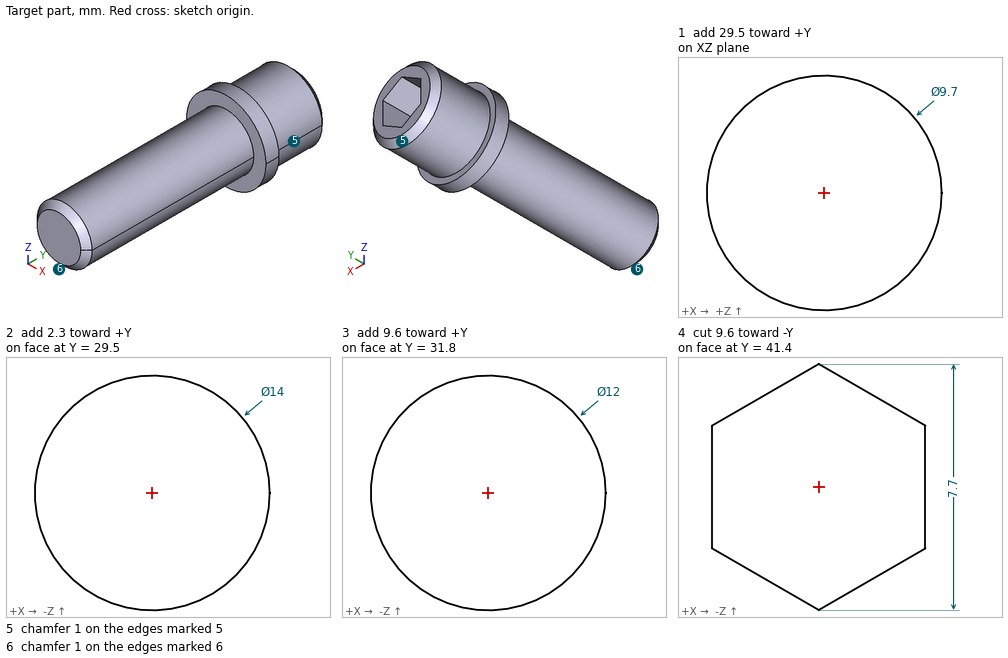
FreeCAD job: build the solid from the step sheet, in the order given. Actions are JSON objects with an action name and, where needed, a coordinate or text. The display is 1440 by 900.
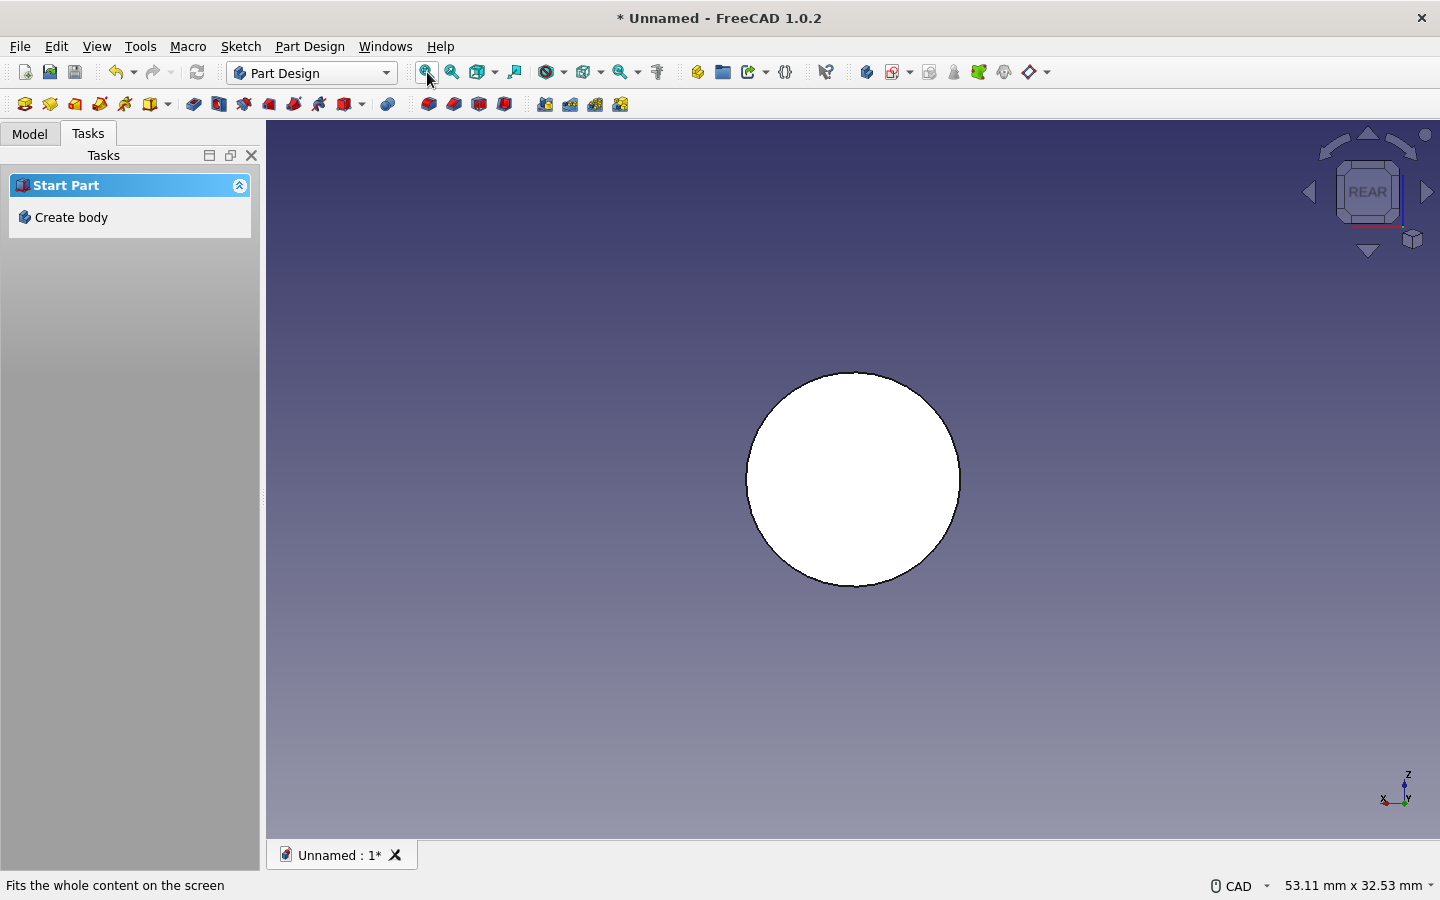
{"action": "left_click", "coordinate": [853, 479]}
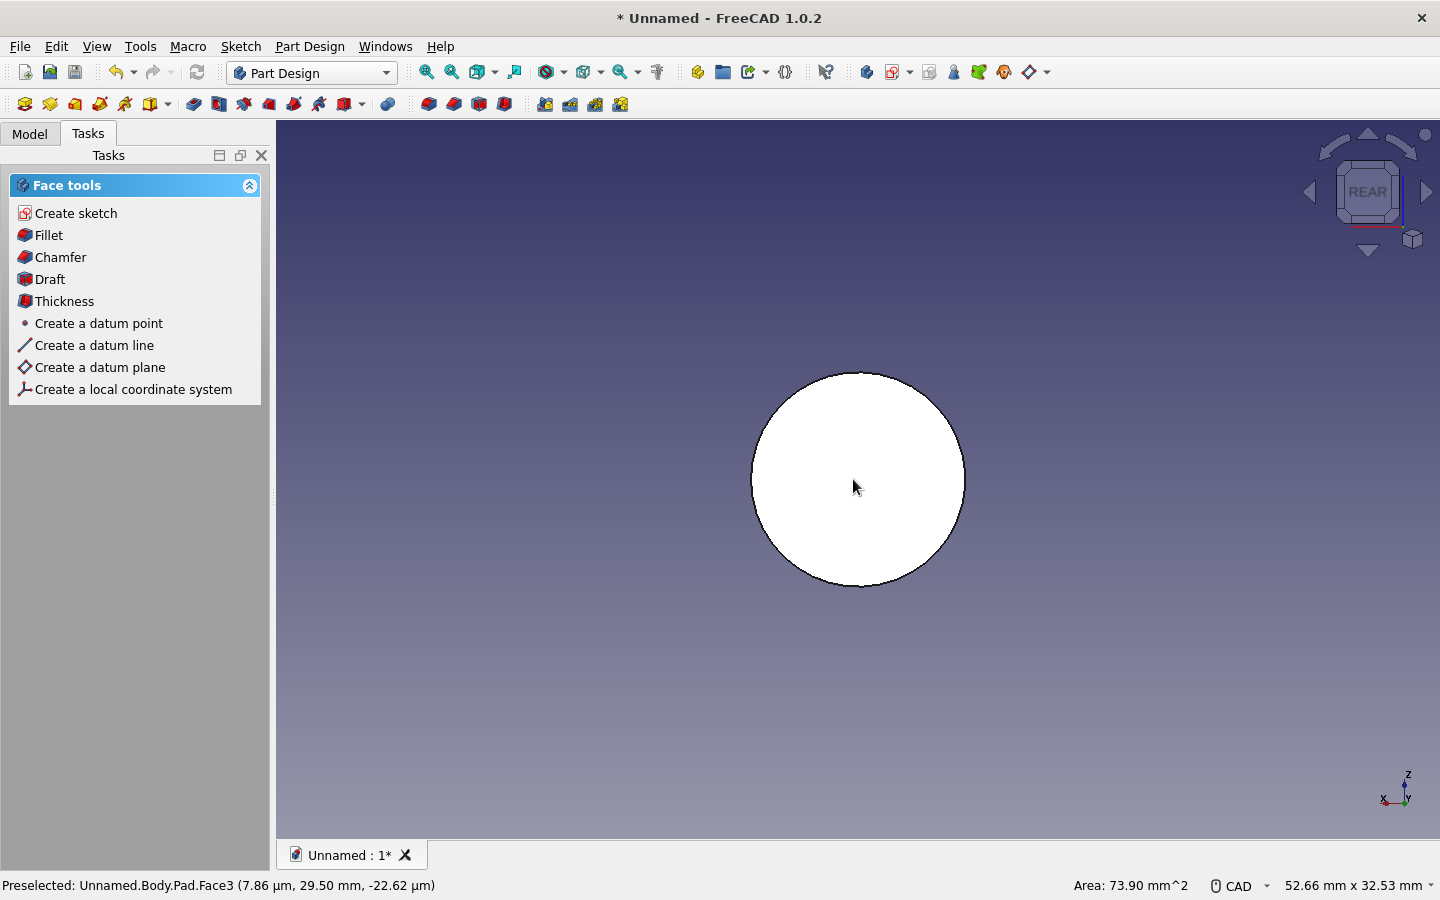
{"action": "left_click", "coordinate": [892, 72]}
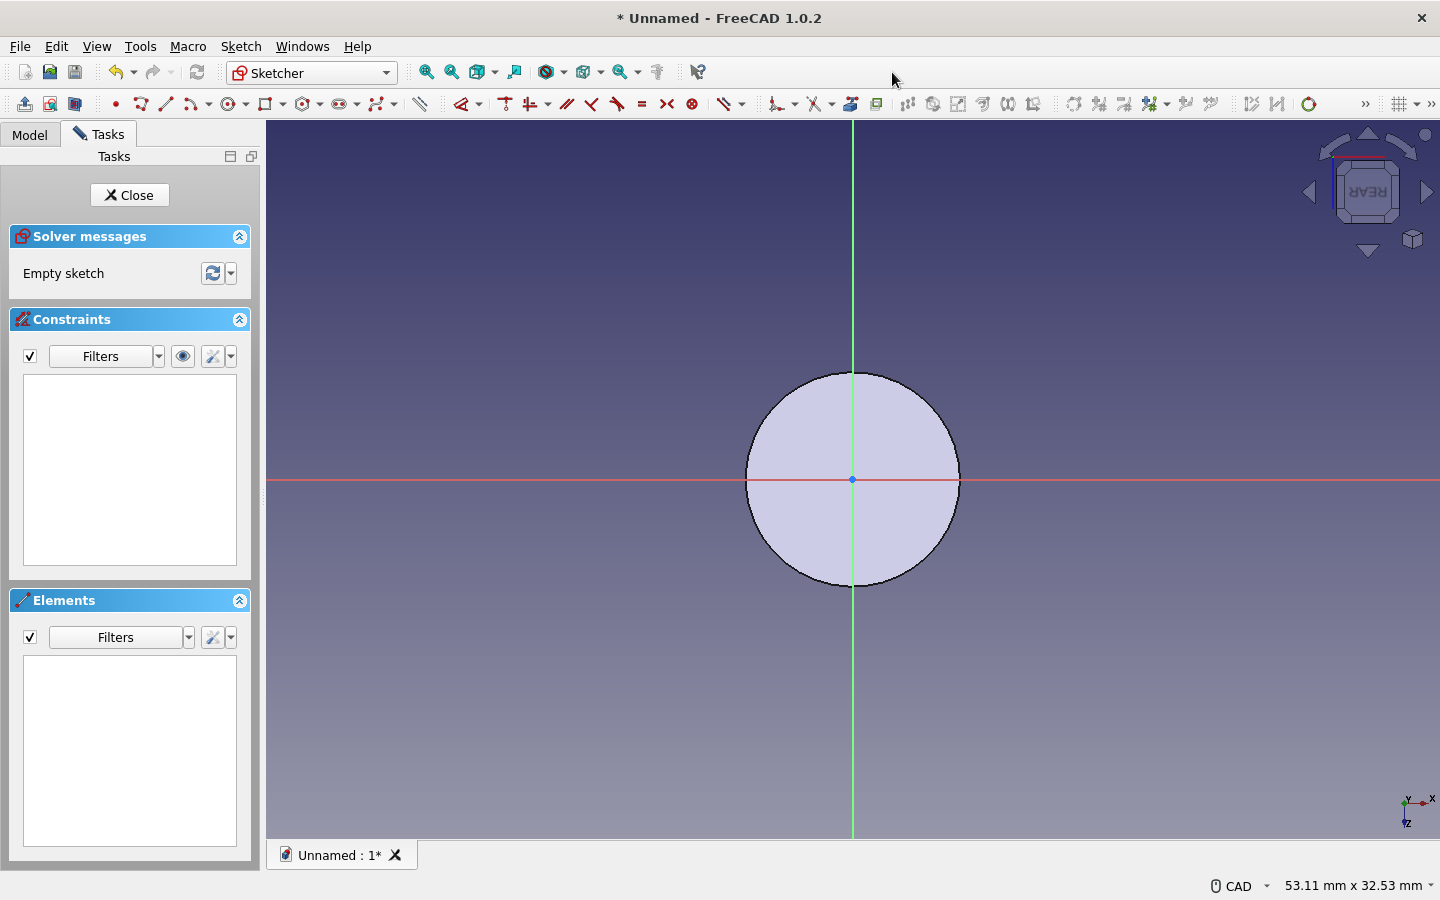
{"action": "scroll", "coordinate": [992, 479], "scroll_direction": "up", "scroll_amount": 2}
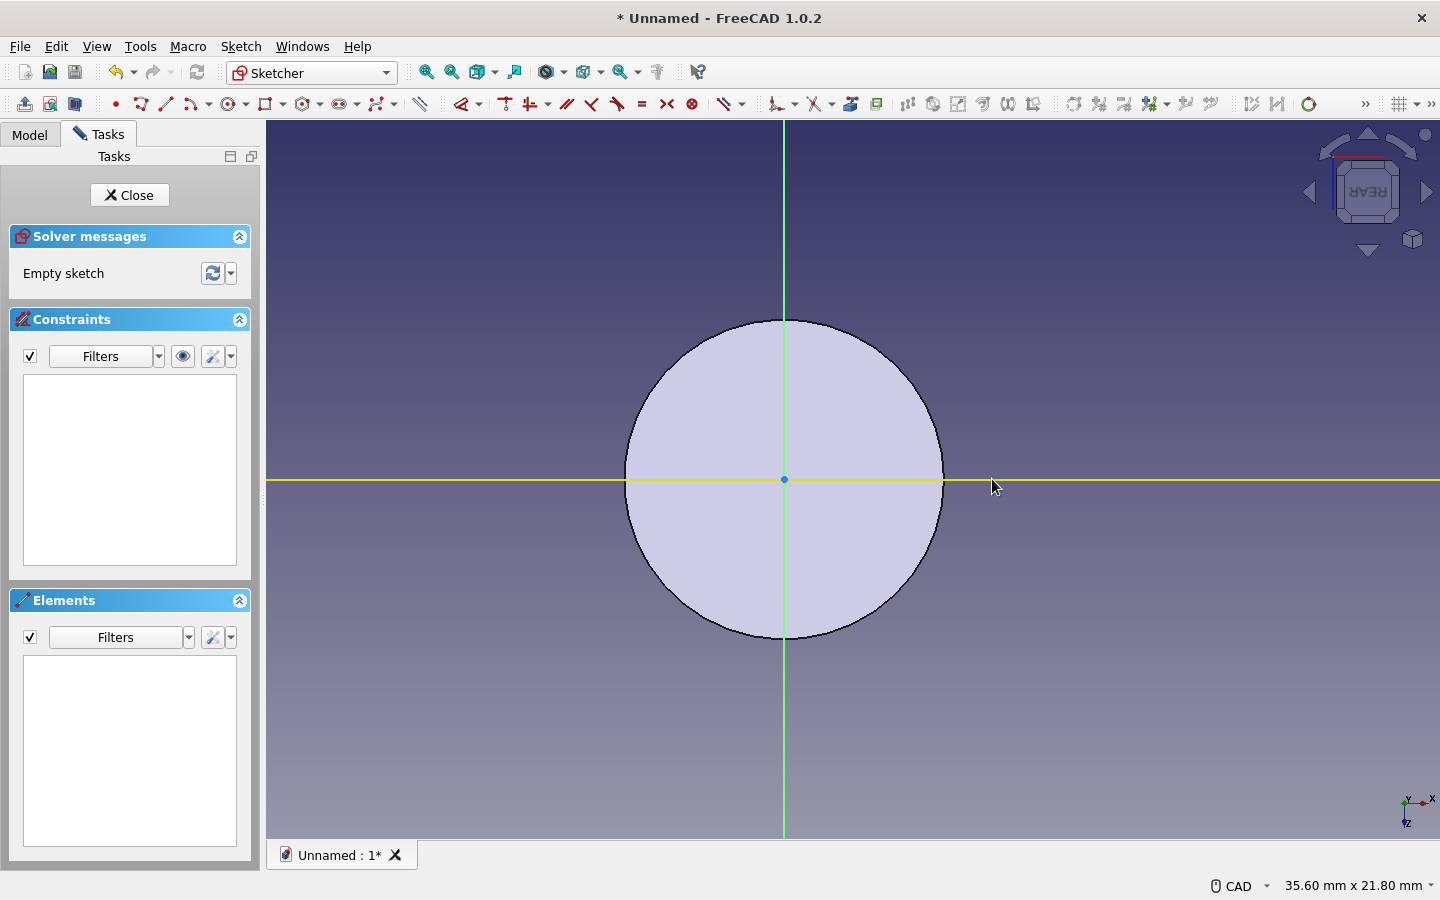
{"action": "left_click", "coordinate": [228, 104]}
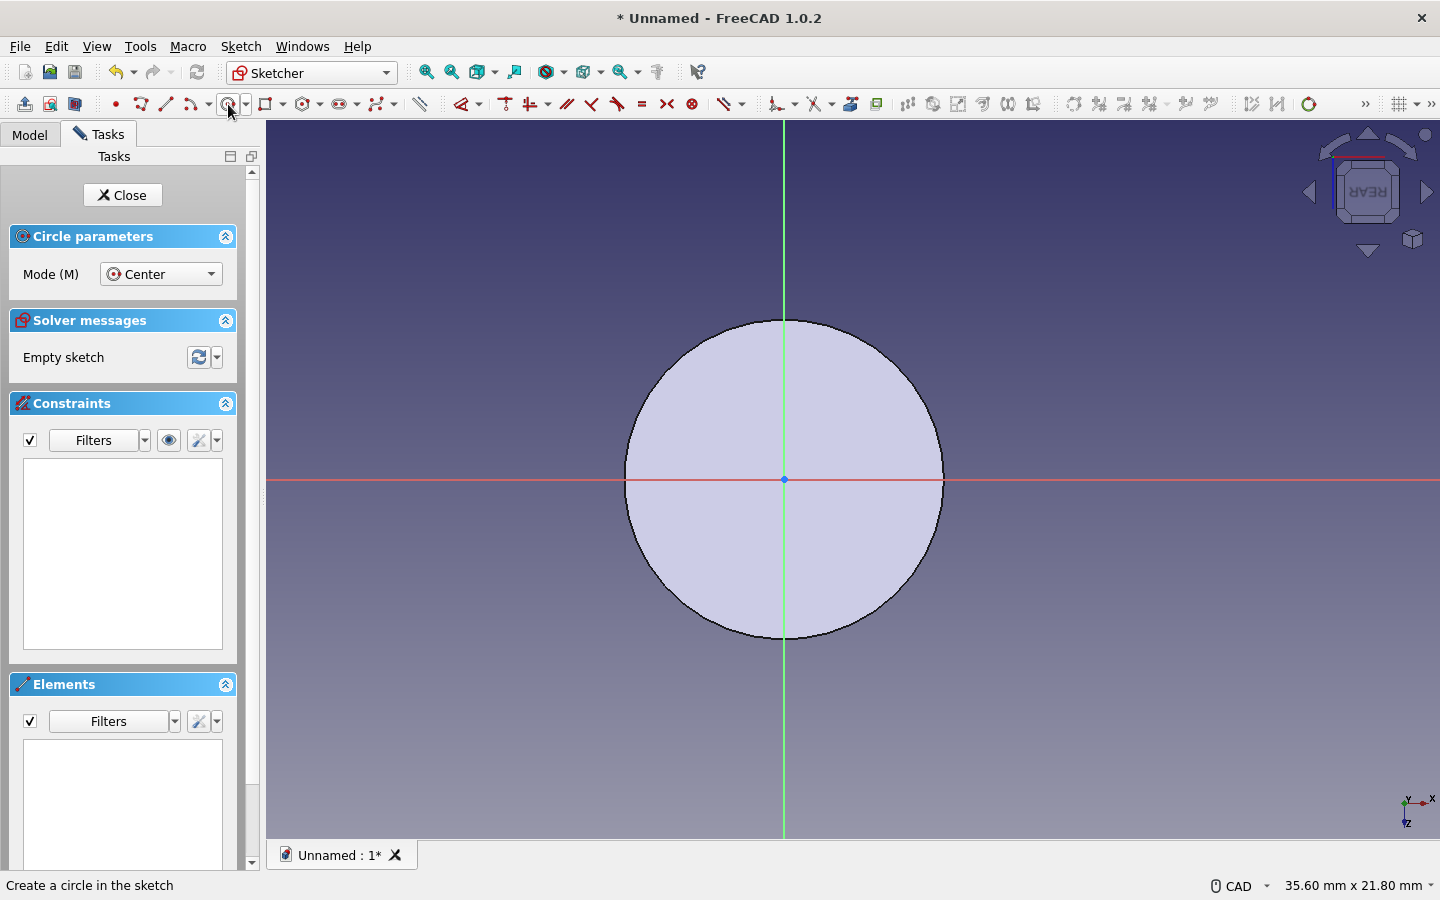
{"action": "left_click", "coordinate": [784, 479]}
{"action": "mouse_move", "coordinate": [947, 316]}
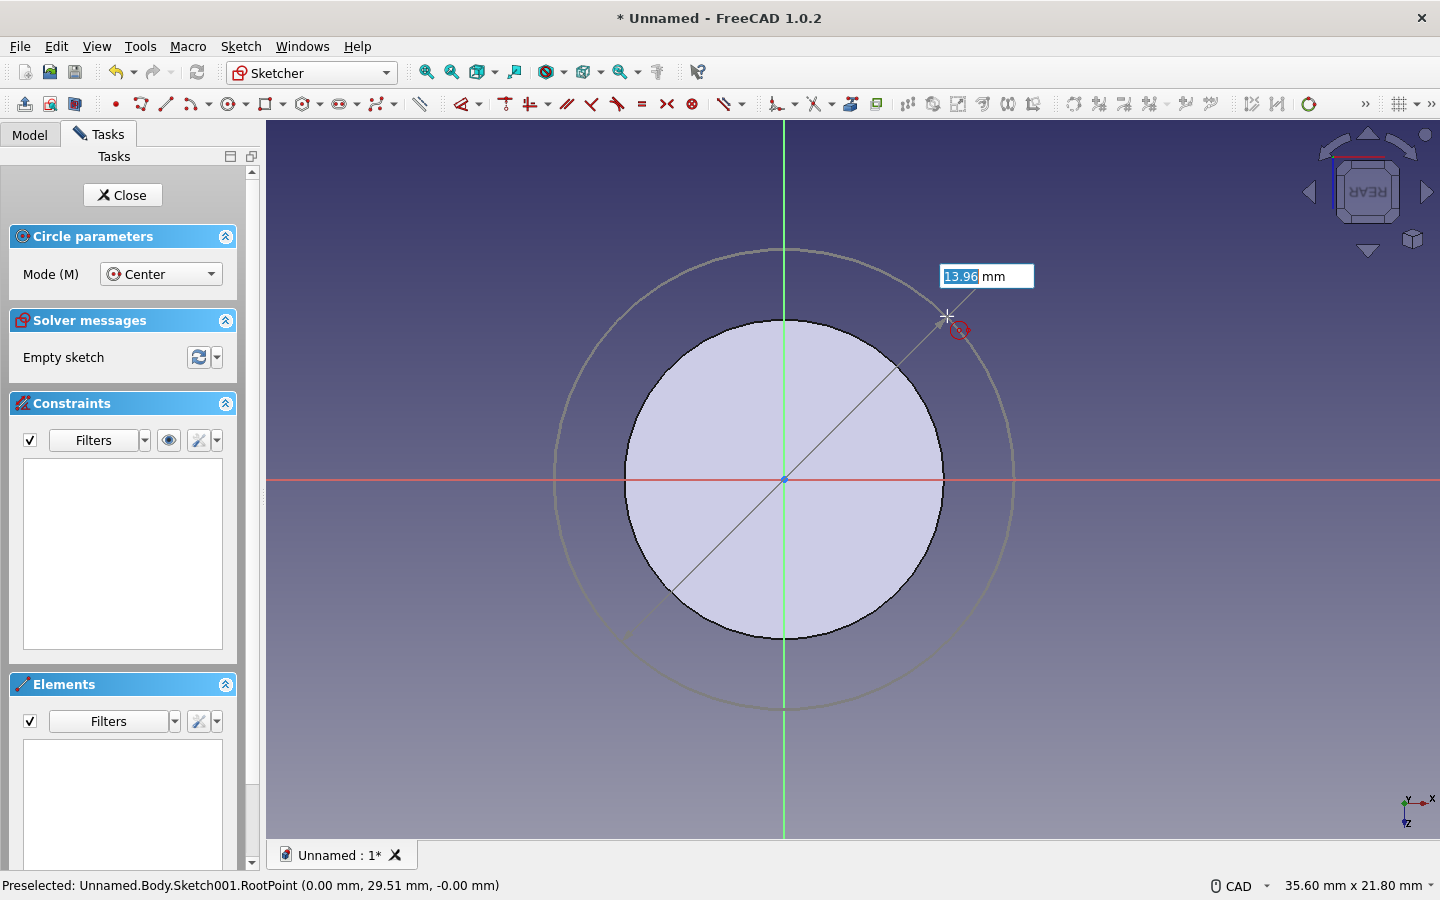
{"action": "type", "text": "14"}
{"action": "key", "text": "Return"}
{"action": "key", "text": "Escape"}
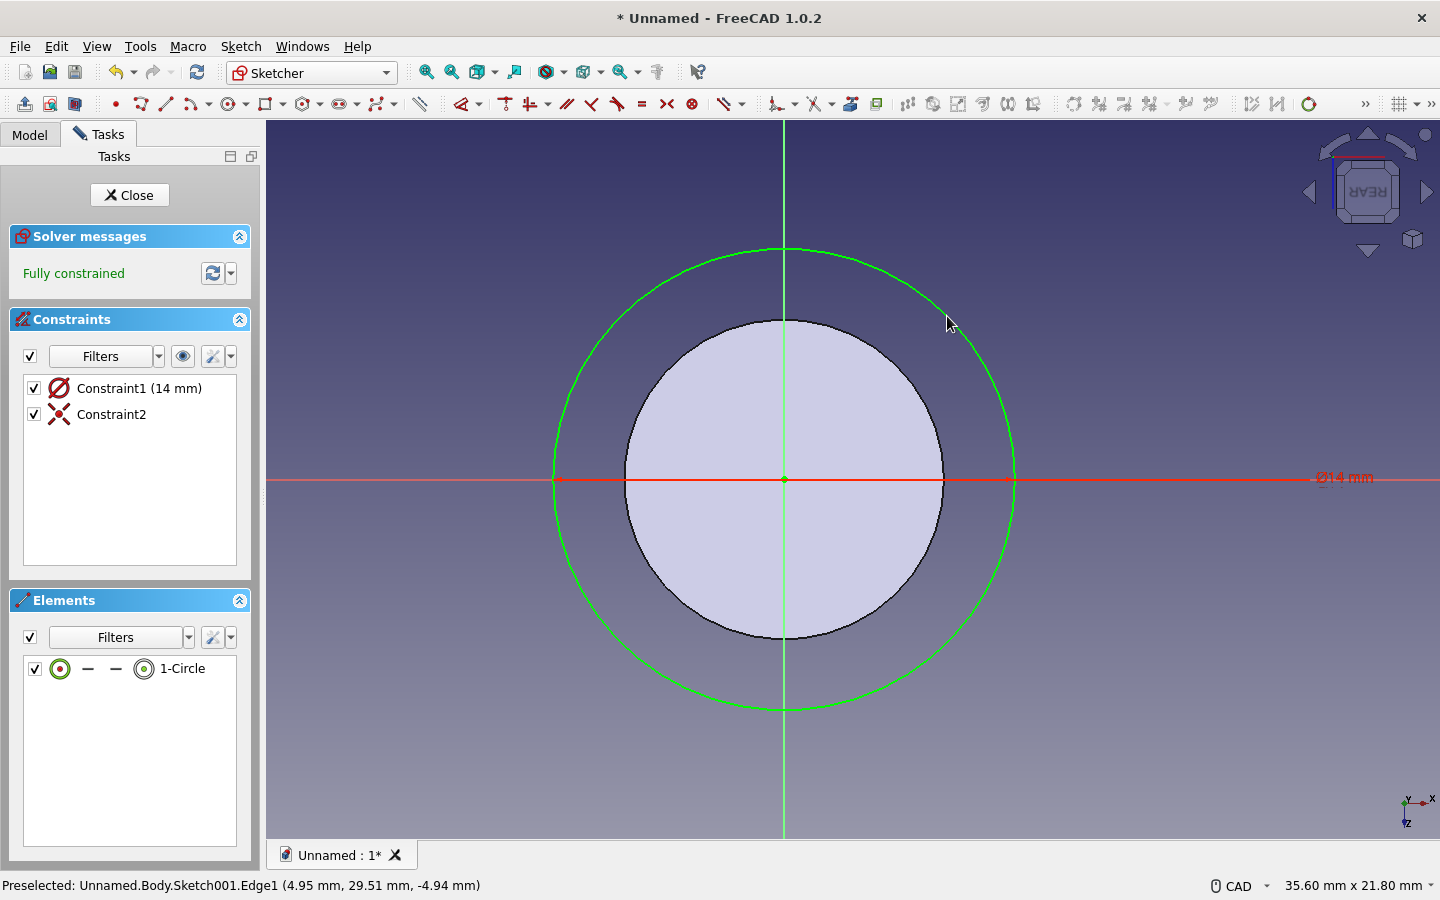
{"action": "left_click", "coordinate": [130, 195]}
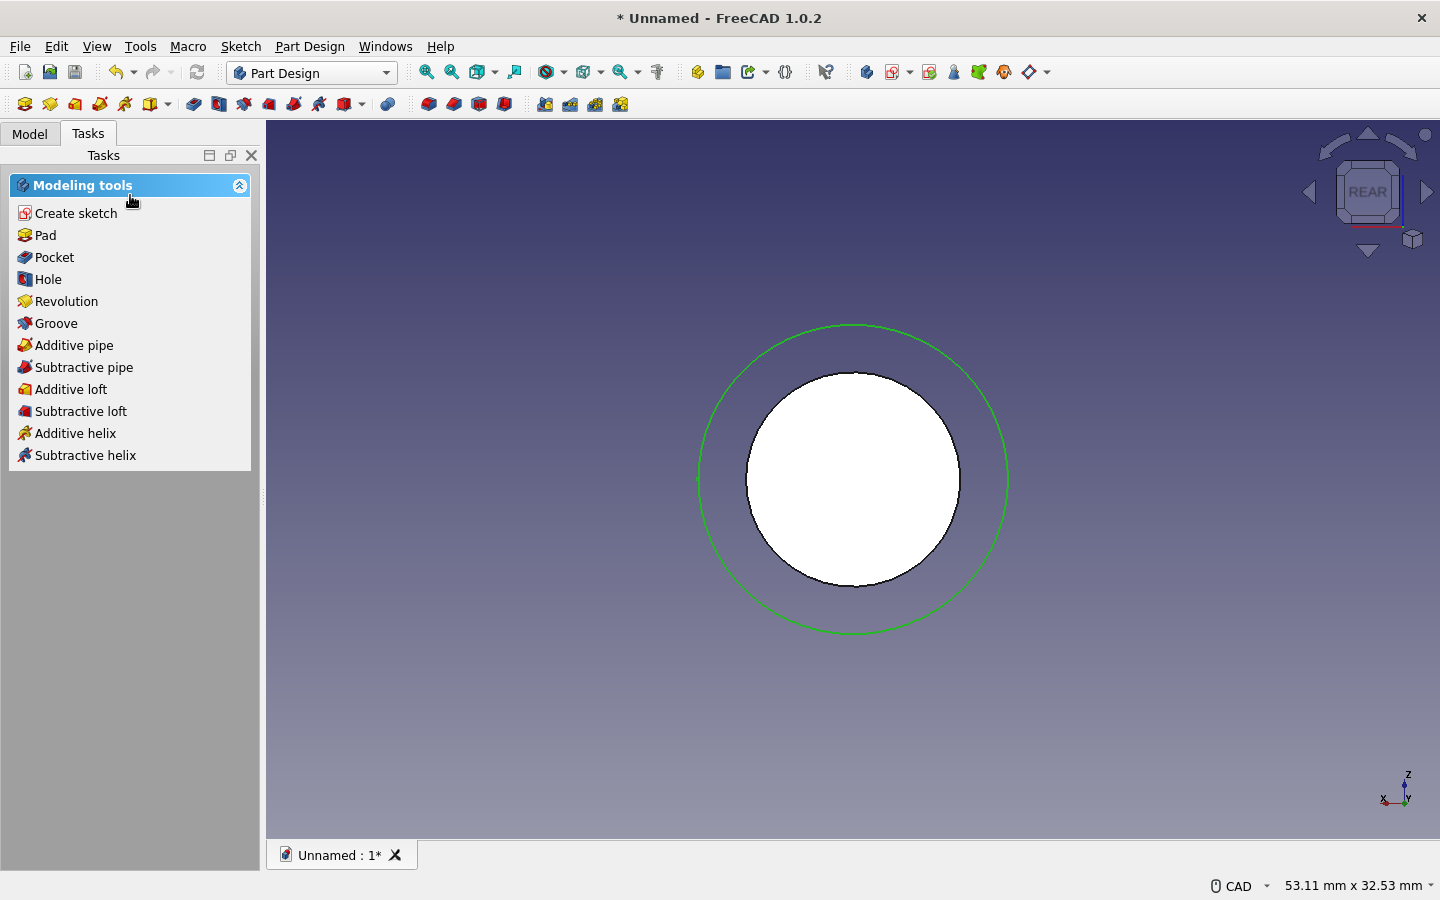
{"action": "left_click", "coordinate": [25, 104]}